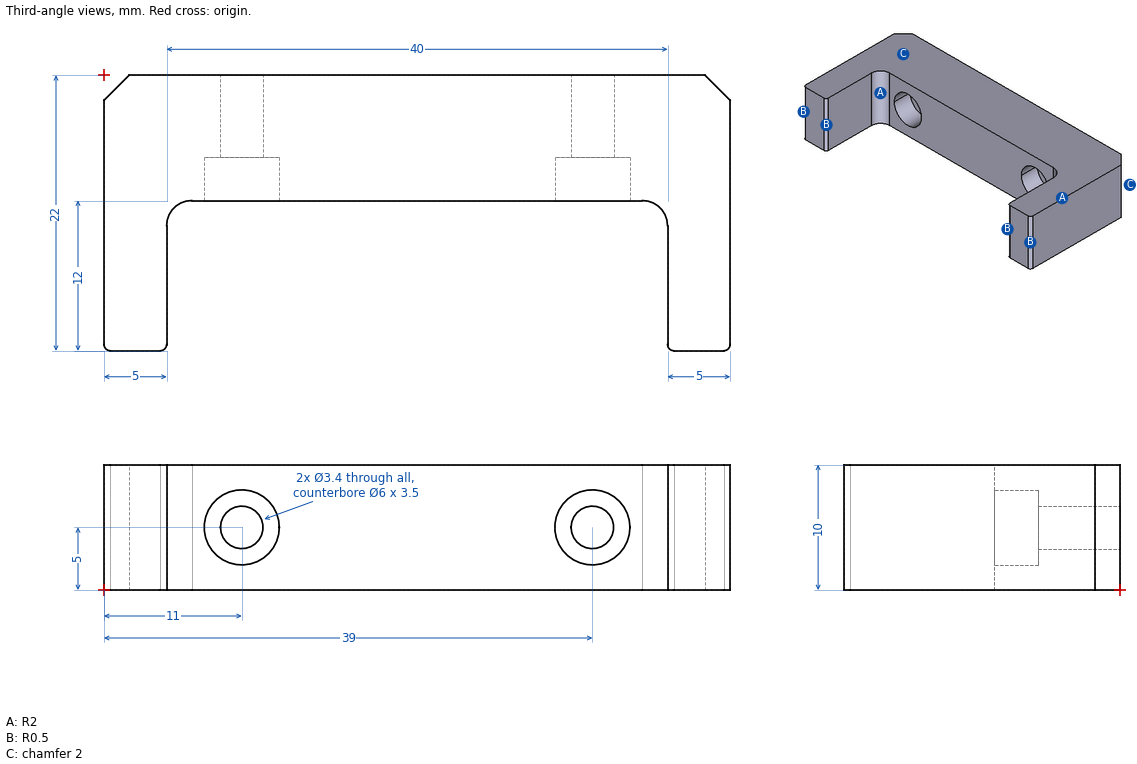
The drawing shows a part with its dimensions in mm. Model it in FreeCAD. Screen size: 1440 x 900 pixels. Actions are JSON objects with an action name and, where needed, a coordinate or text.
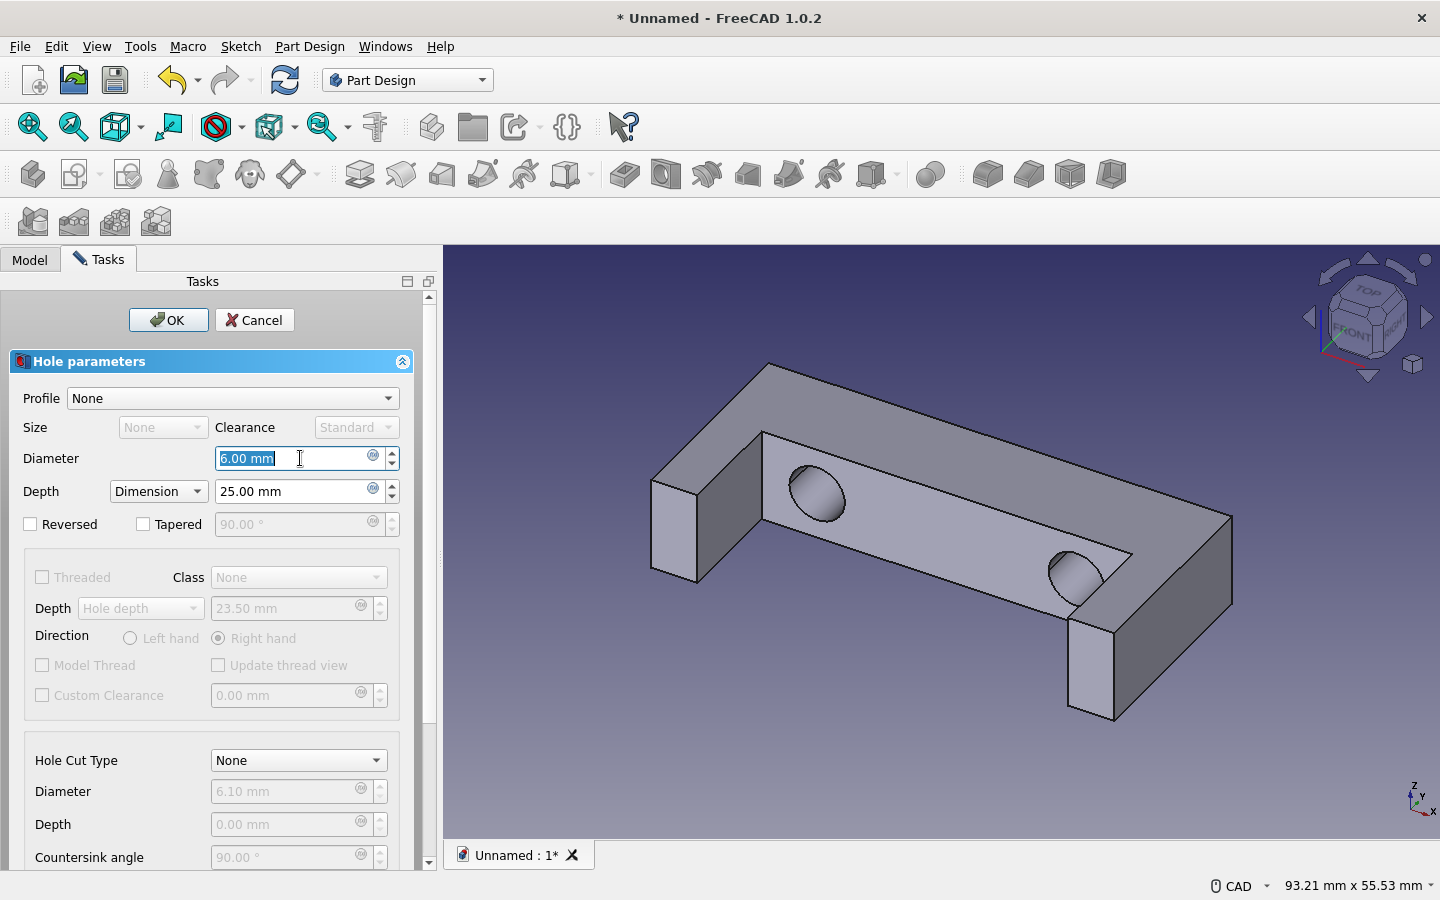
{"action": "type", "text": "3.4"}
{"action": "key", "text": "Tab"}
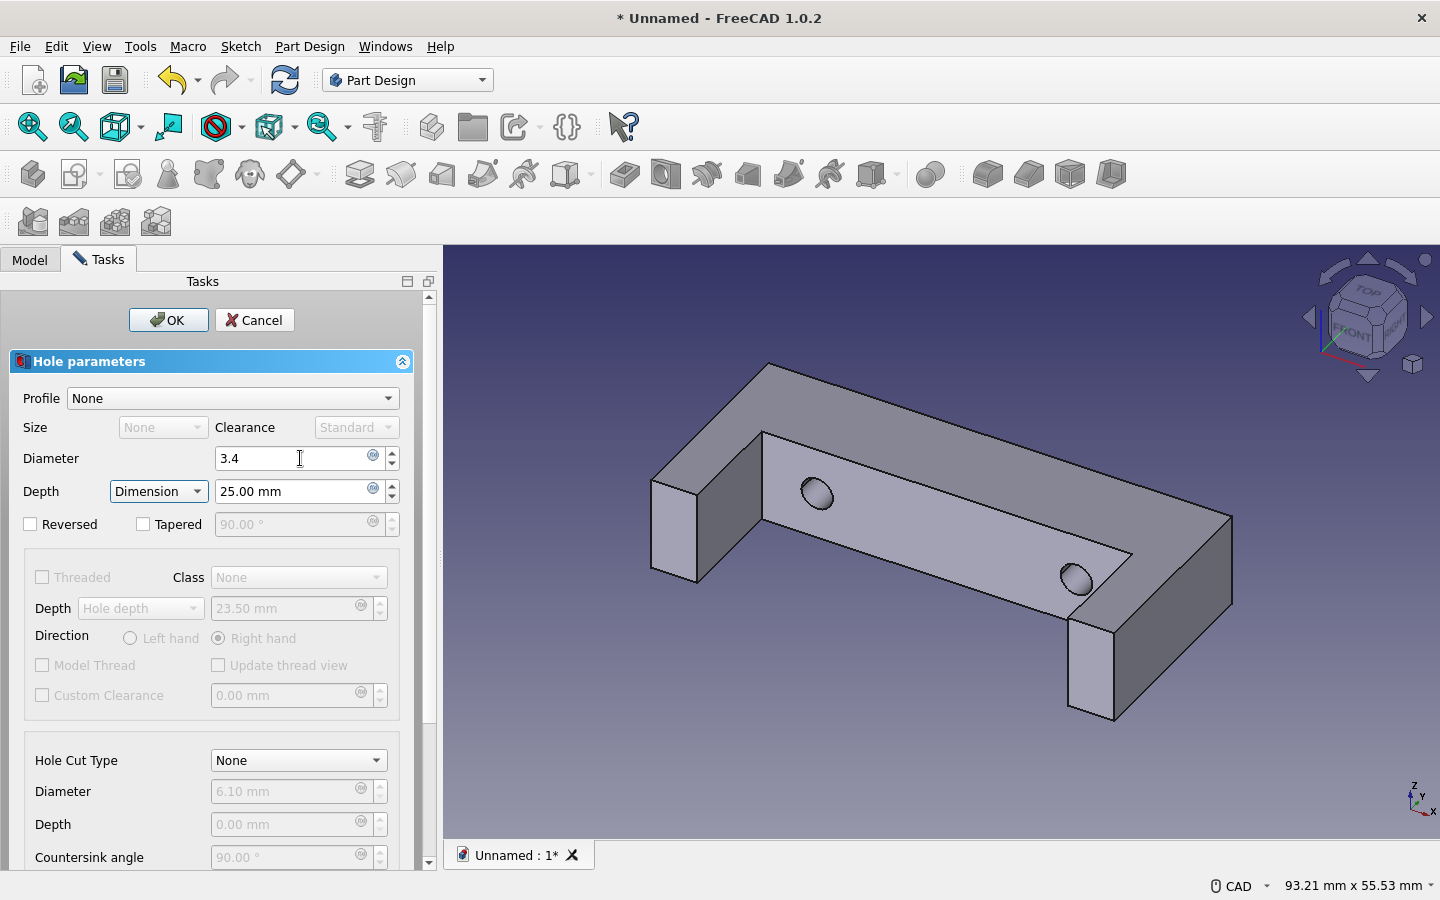
{"action": "left_click", "coordinate": [160, 492]}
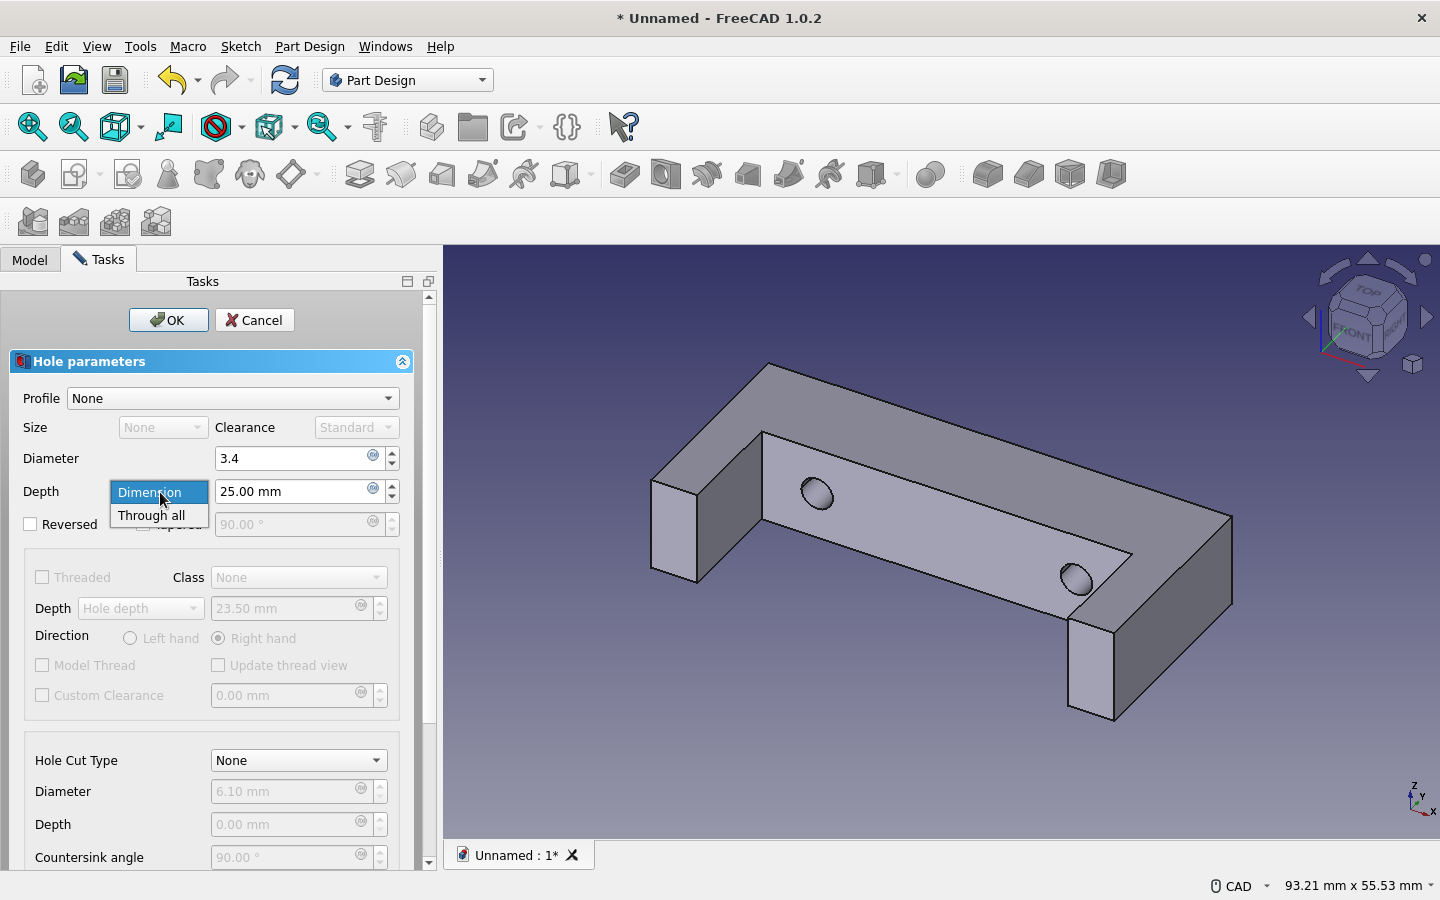
{"action": "left_click", "coordinate": [158, 516]}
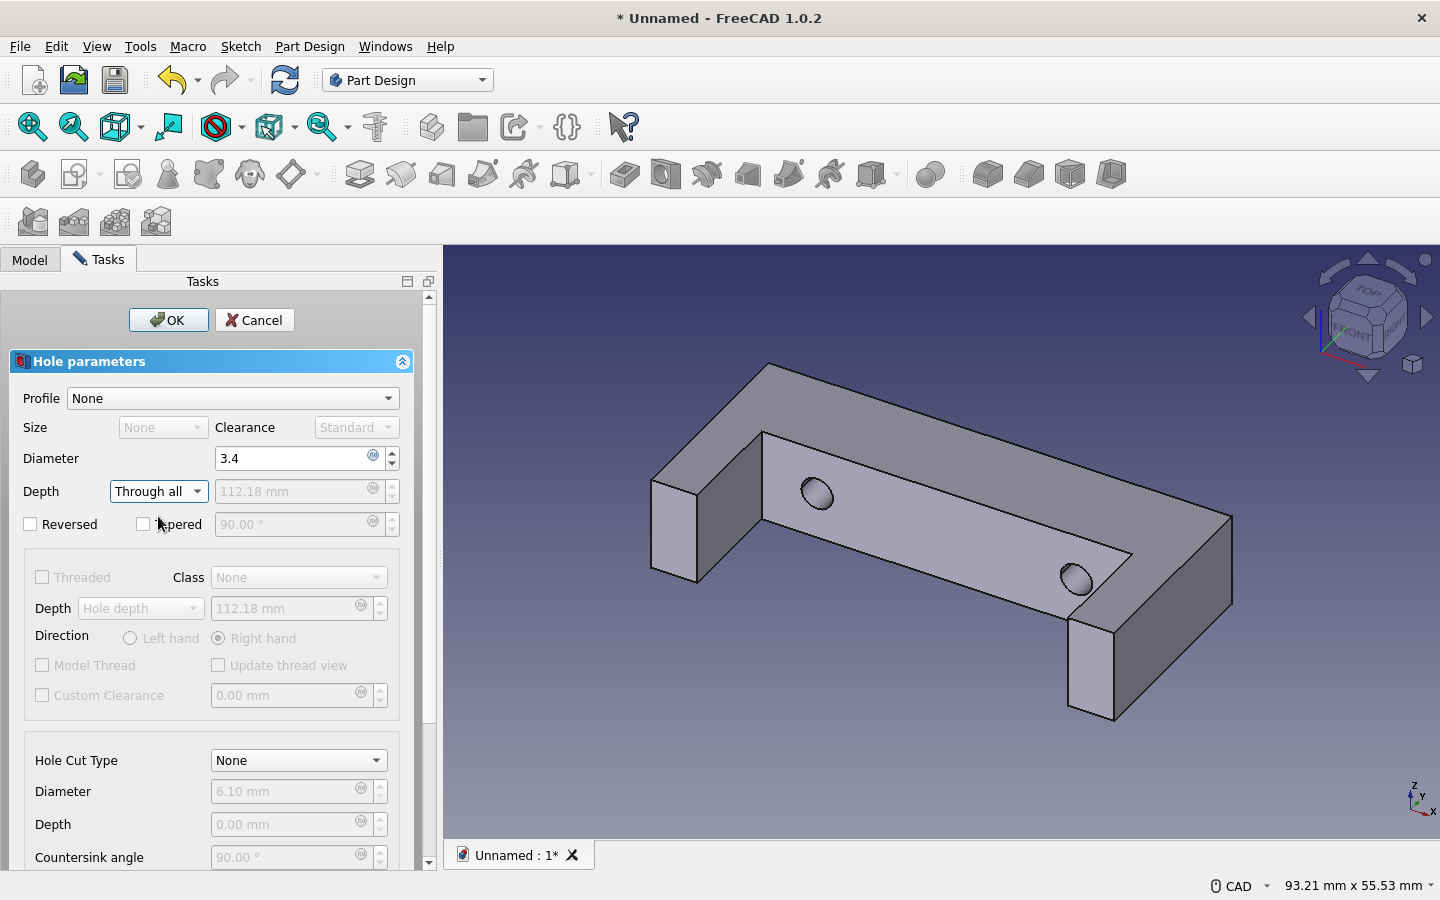
{"action": "left_click", "coordinate": [300, 760]}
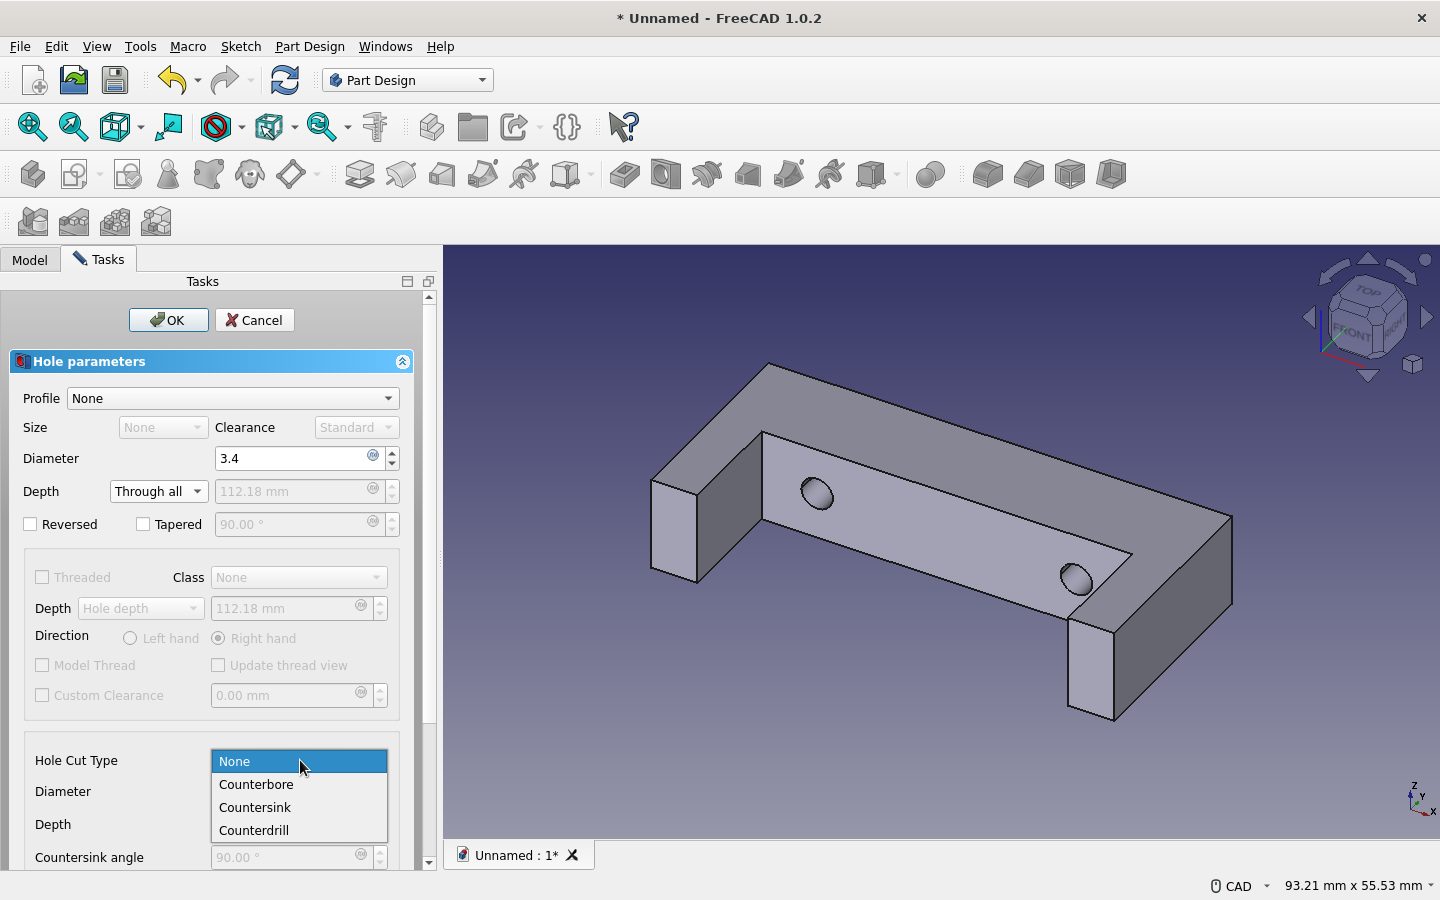
{"action": "left_click", "coordinate": [298, 784]}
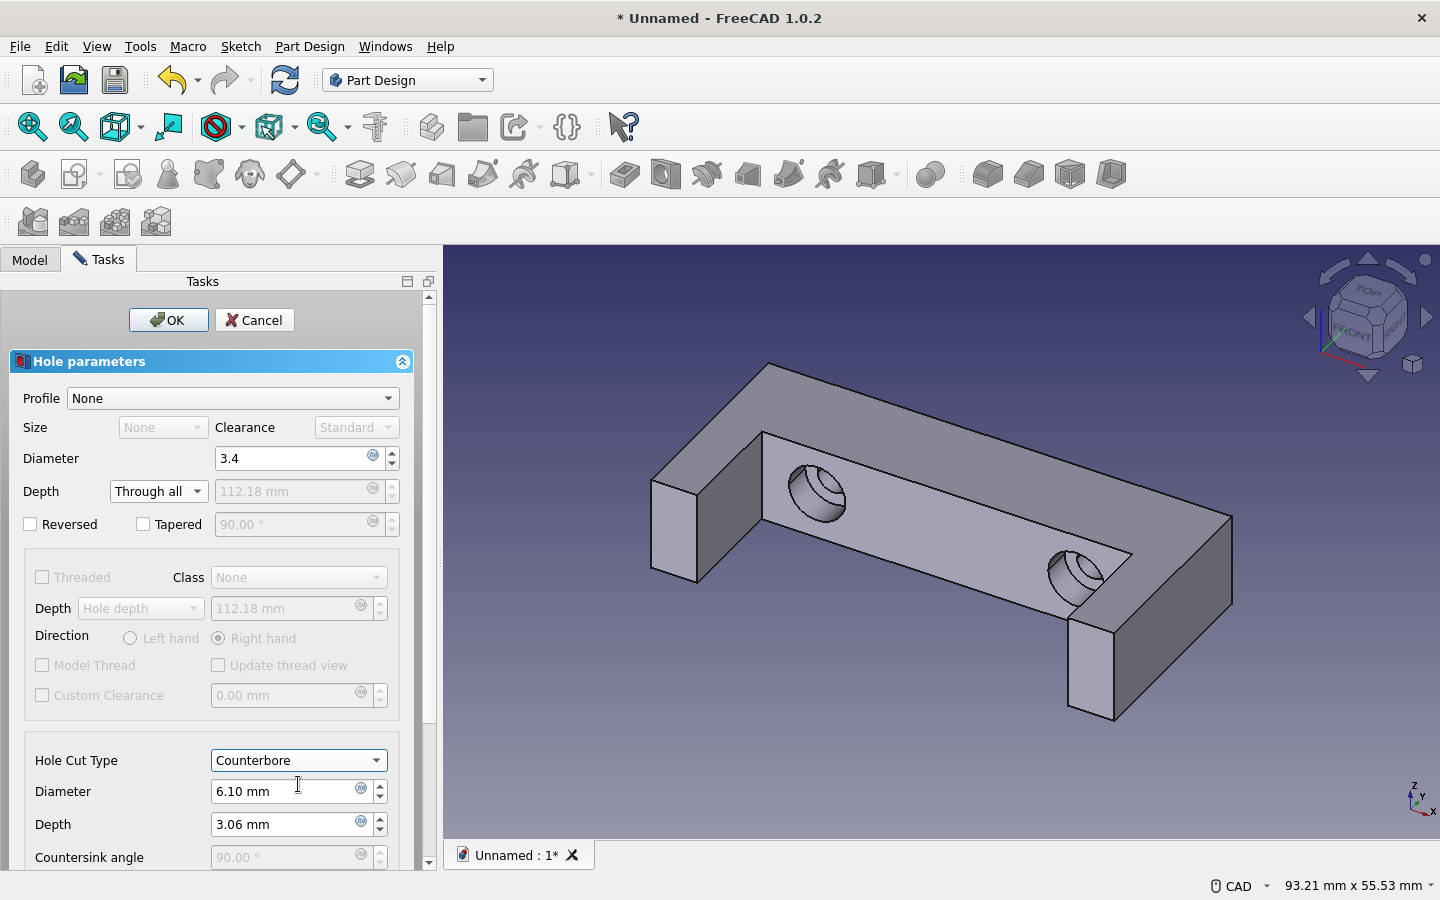
{"action": "triple_click", "coordinate": [292, 792]}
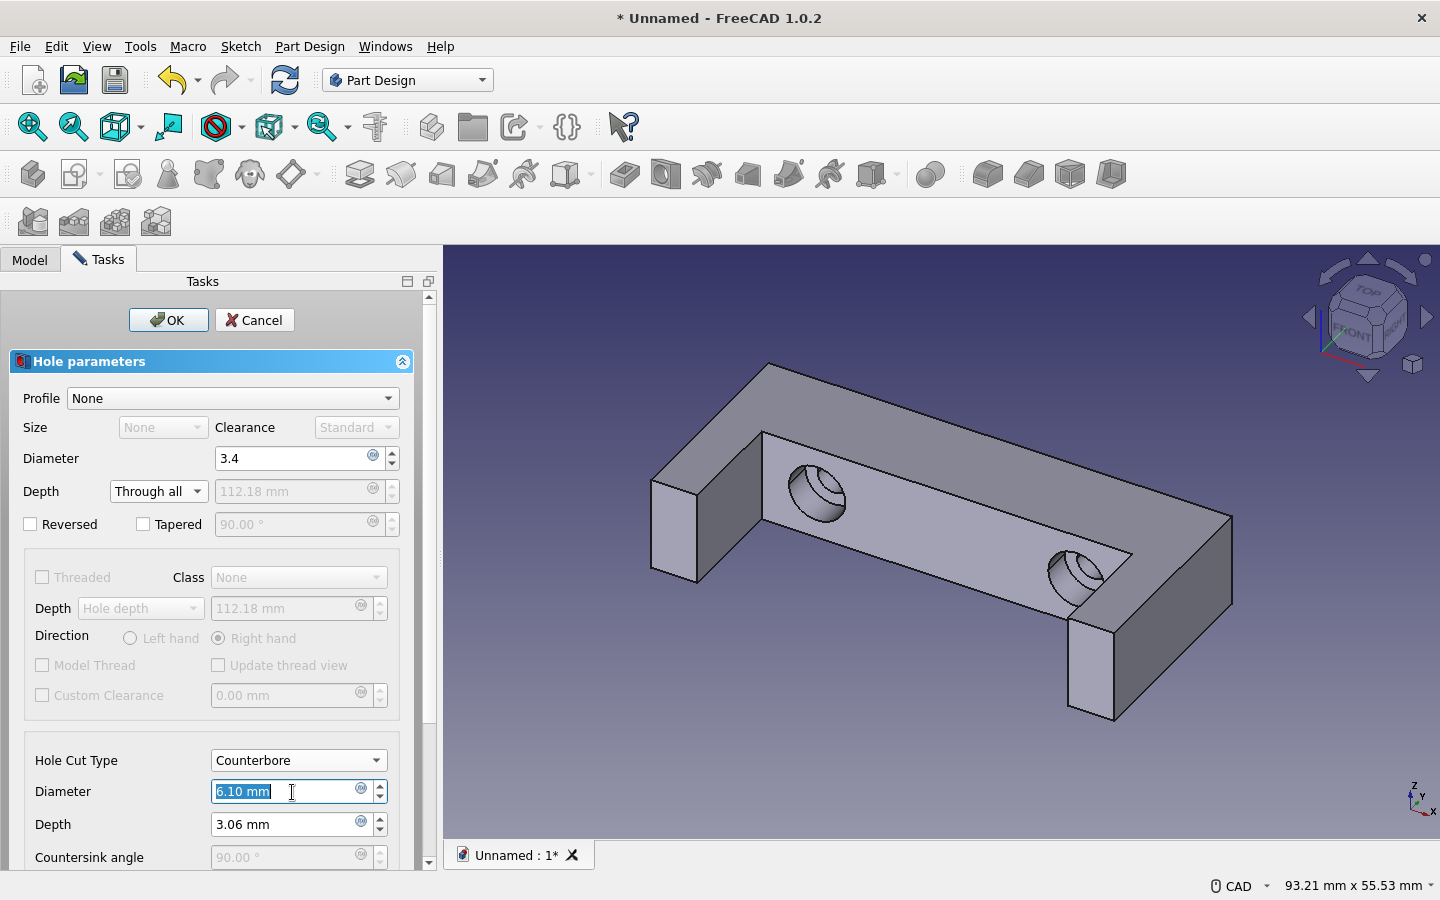
{"action": "type", "text": "6"}
{"action": "key", "text": "Tab"}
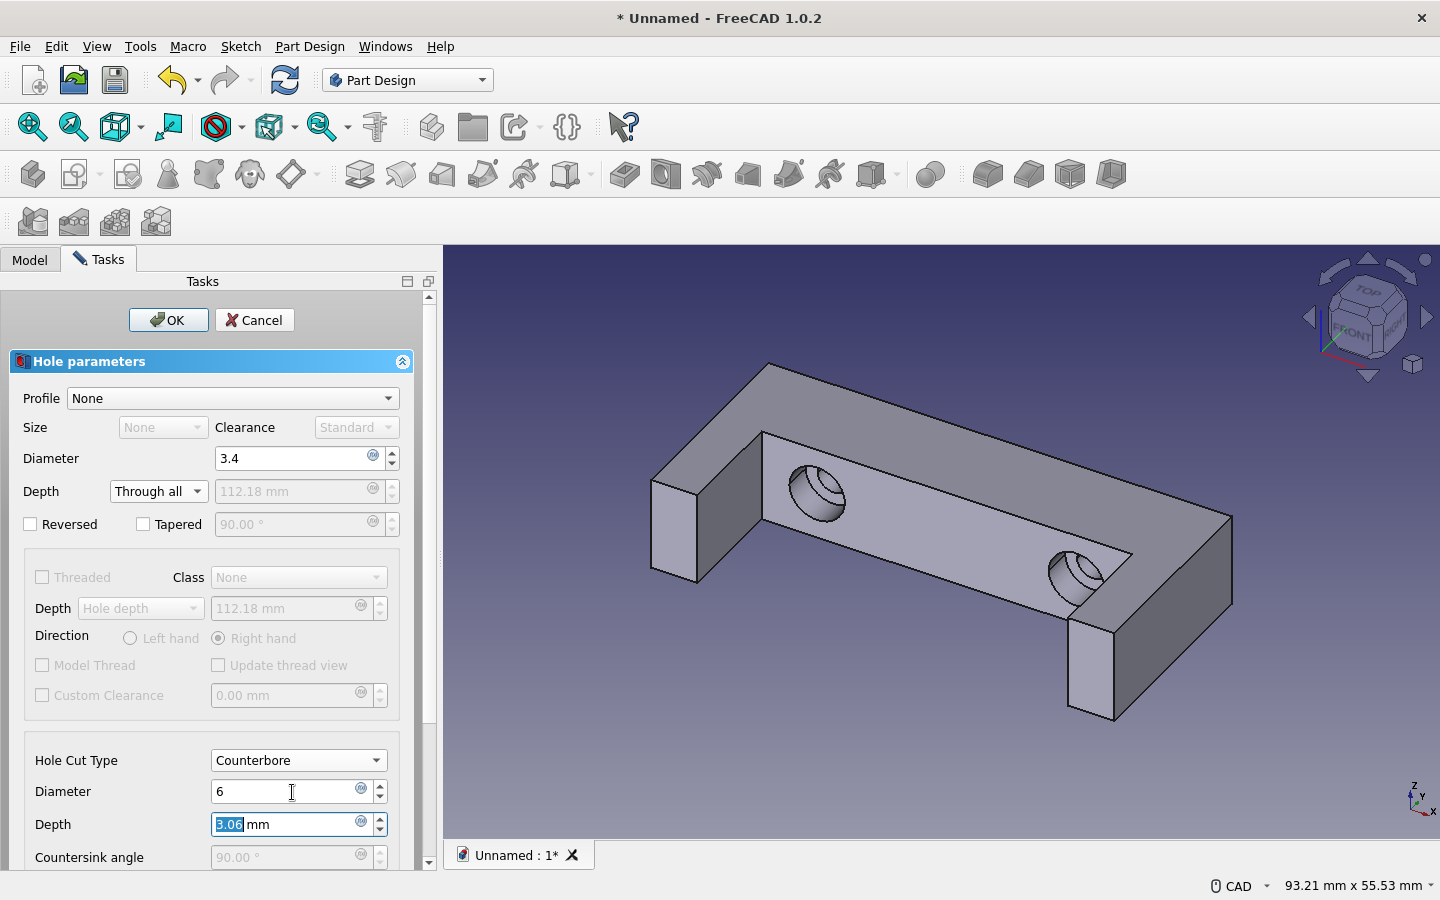
{"action": "type", "text": "3.5"}
{"action": "key", "text": "Tab"}